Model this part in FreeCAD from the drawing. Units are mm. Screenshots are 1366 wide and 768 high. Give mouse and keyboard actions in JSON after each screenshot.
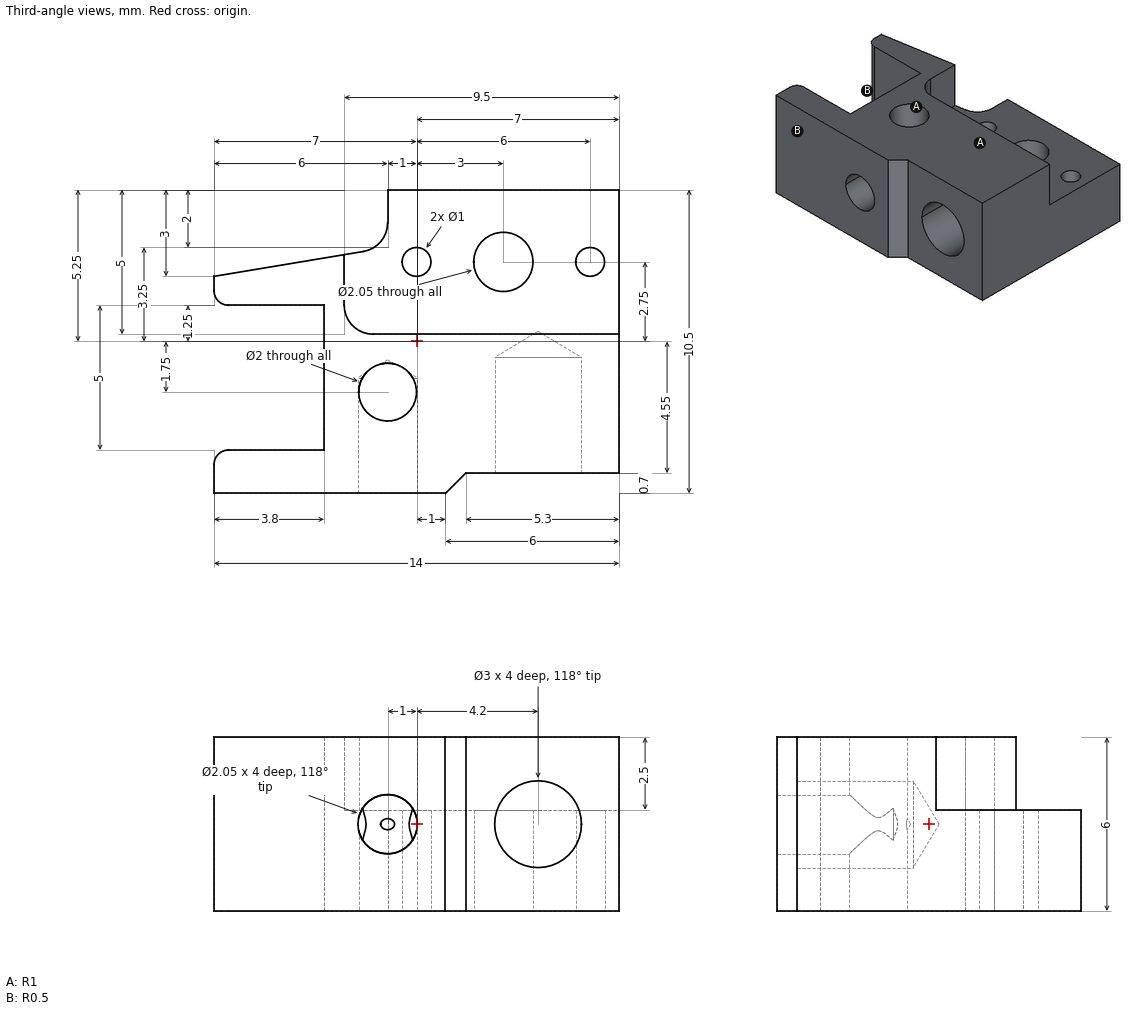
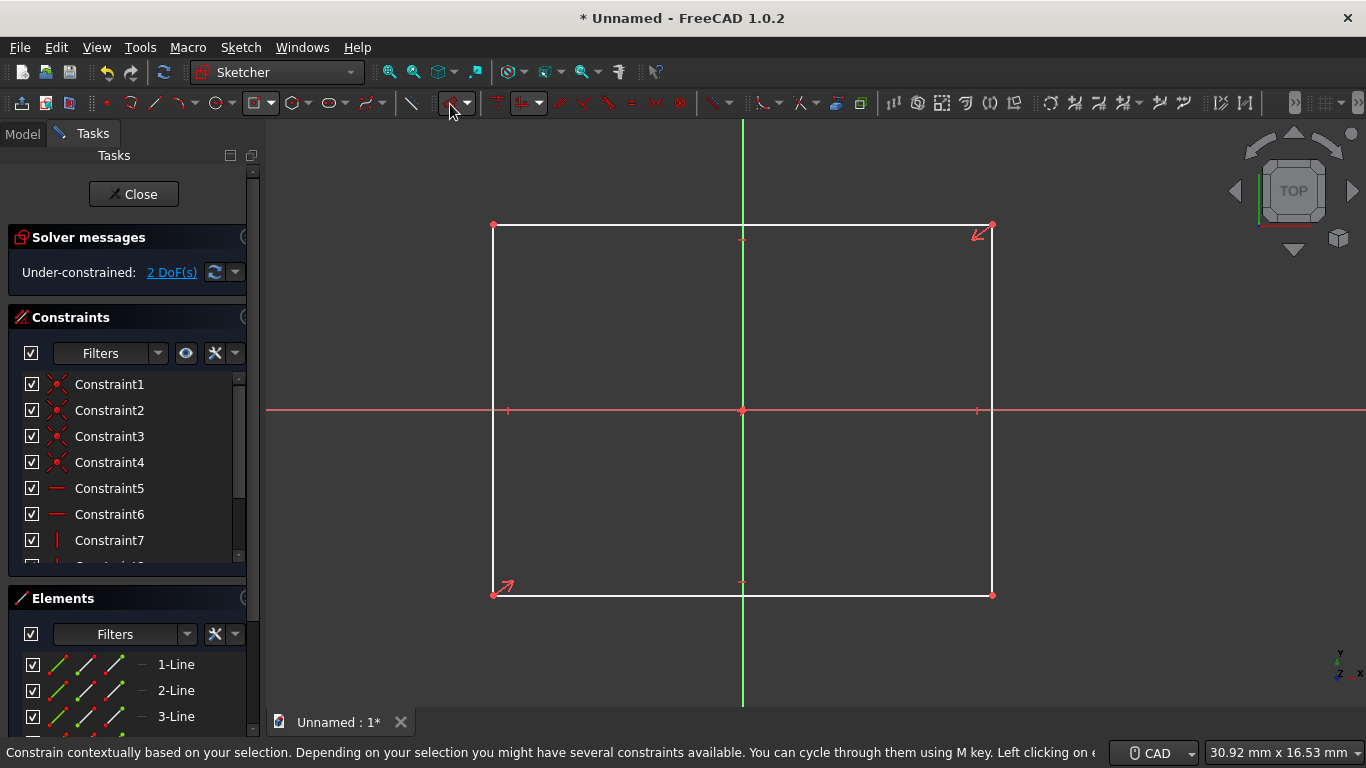
{"action": "left_click", "coordinate": [643, 596]}
{"action": "left_click", "coordinate": [628, 630]}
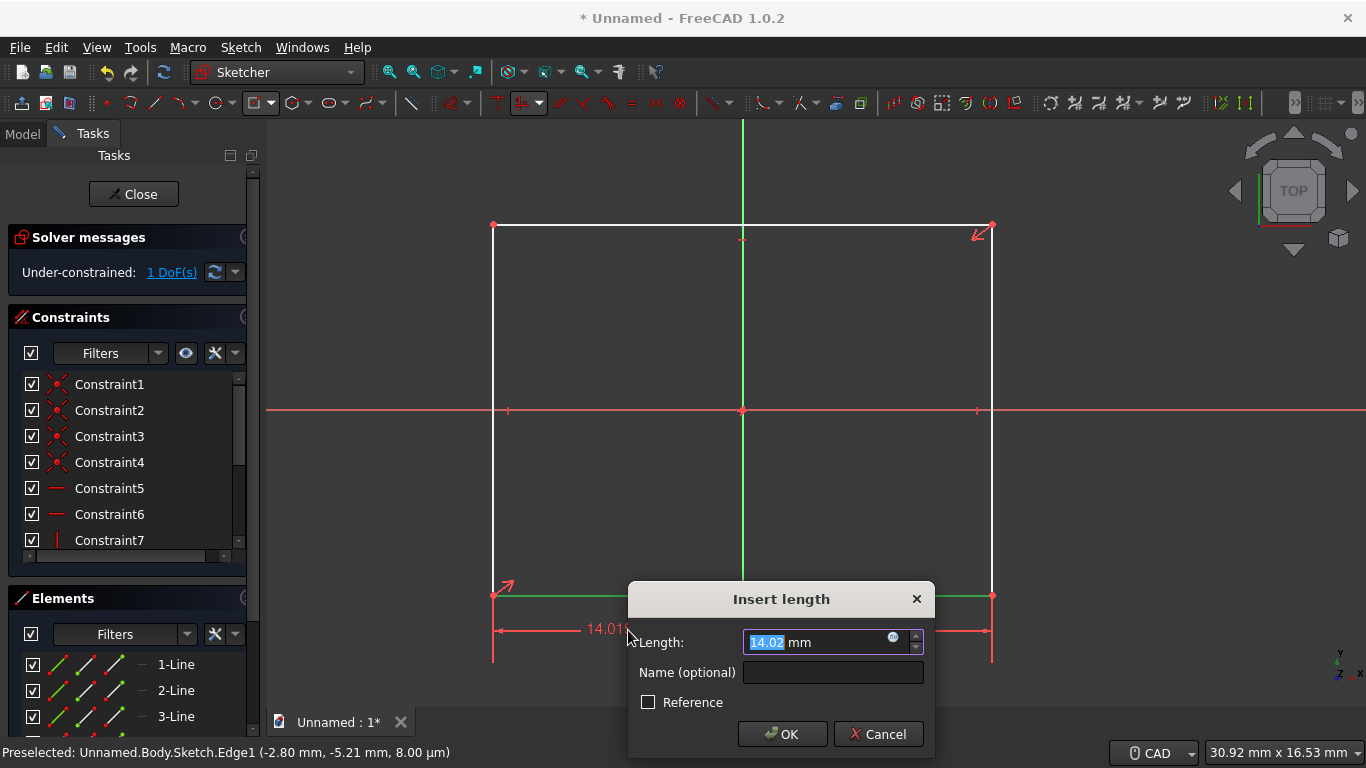
{"action": "type", "text": "14"}
{"action": "key", "text": "Return"}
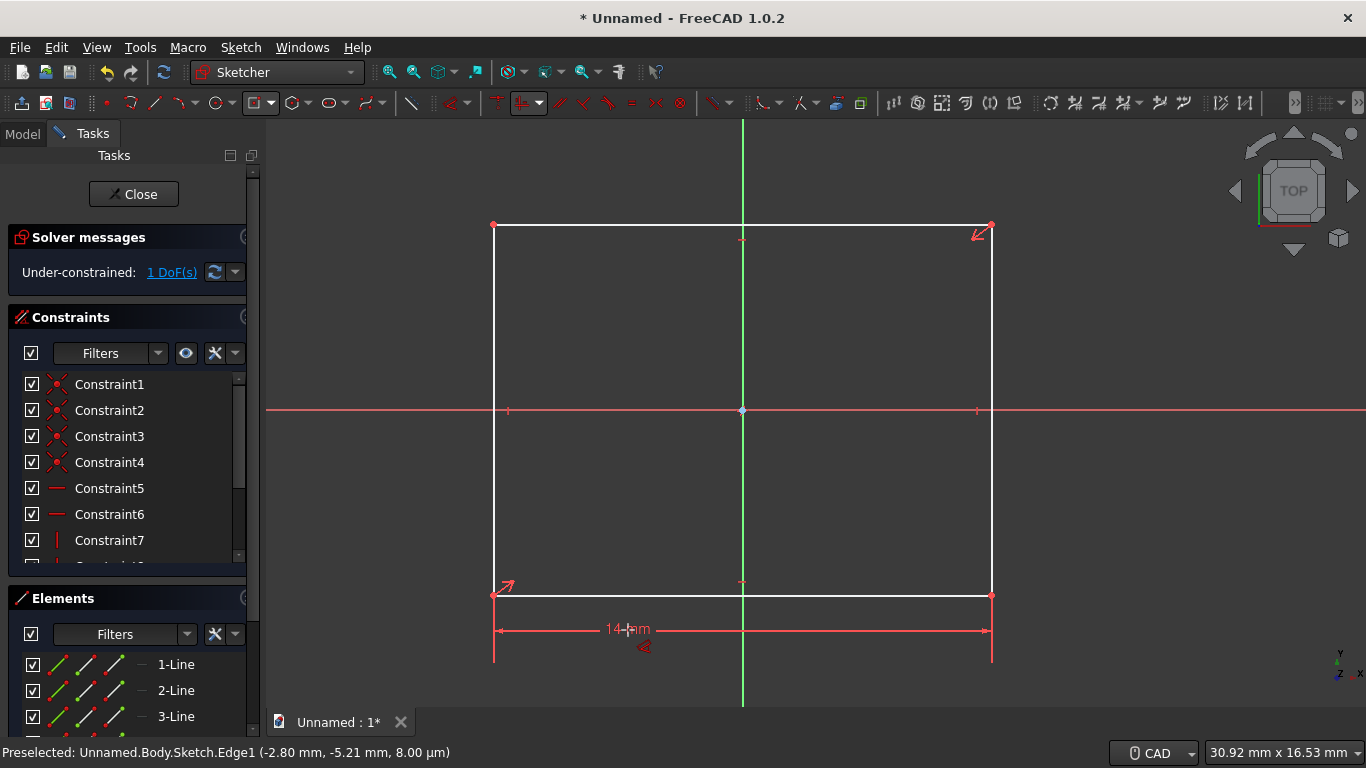
{"action": "left_click", "coordinate": [992, 485]}
{"action": "left_click", "coordinate": [1026, 325]}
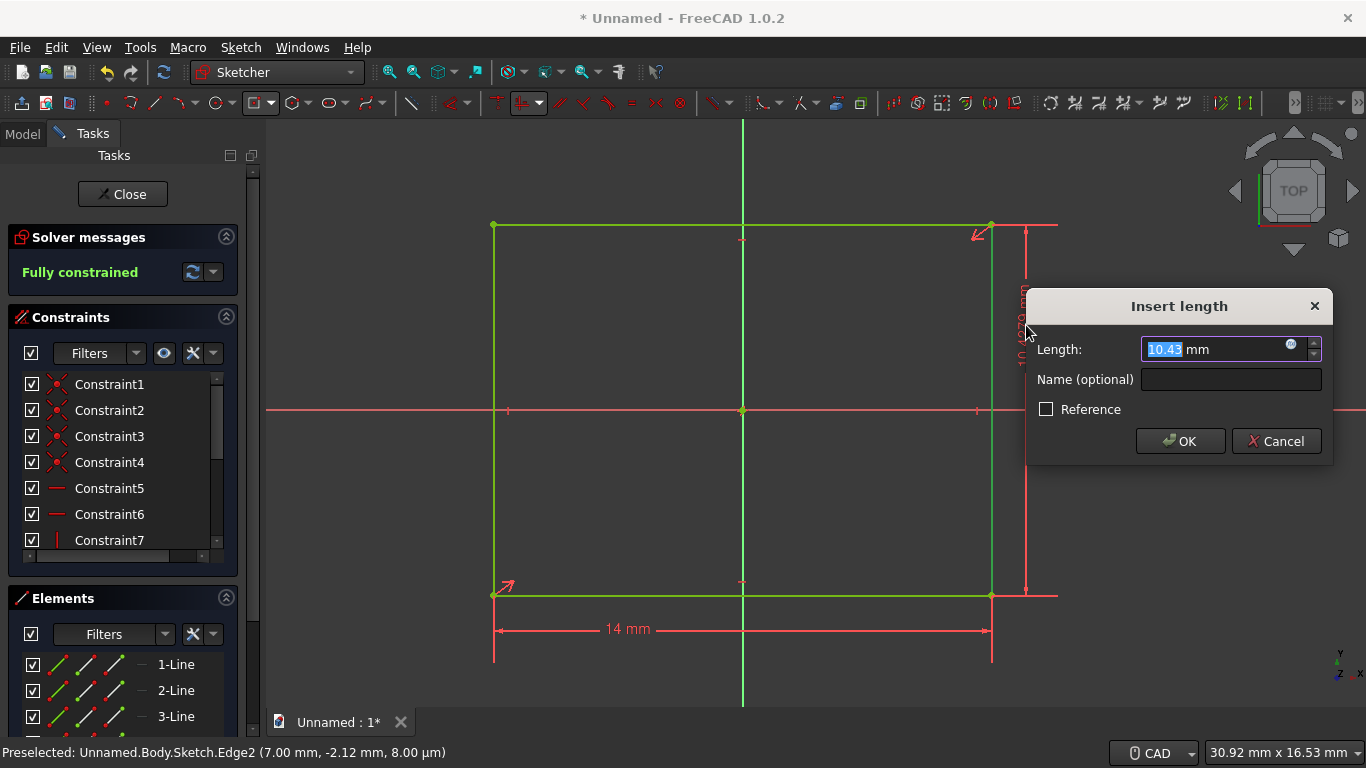
{"action": "type", "text": "10.5"}
{"action": "key", "text": "Return"}
{"action": "key", "text": "Escape"}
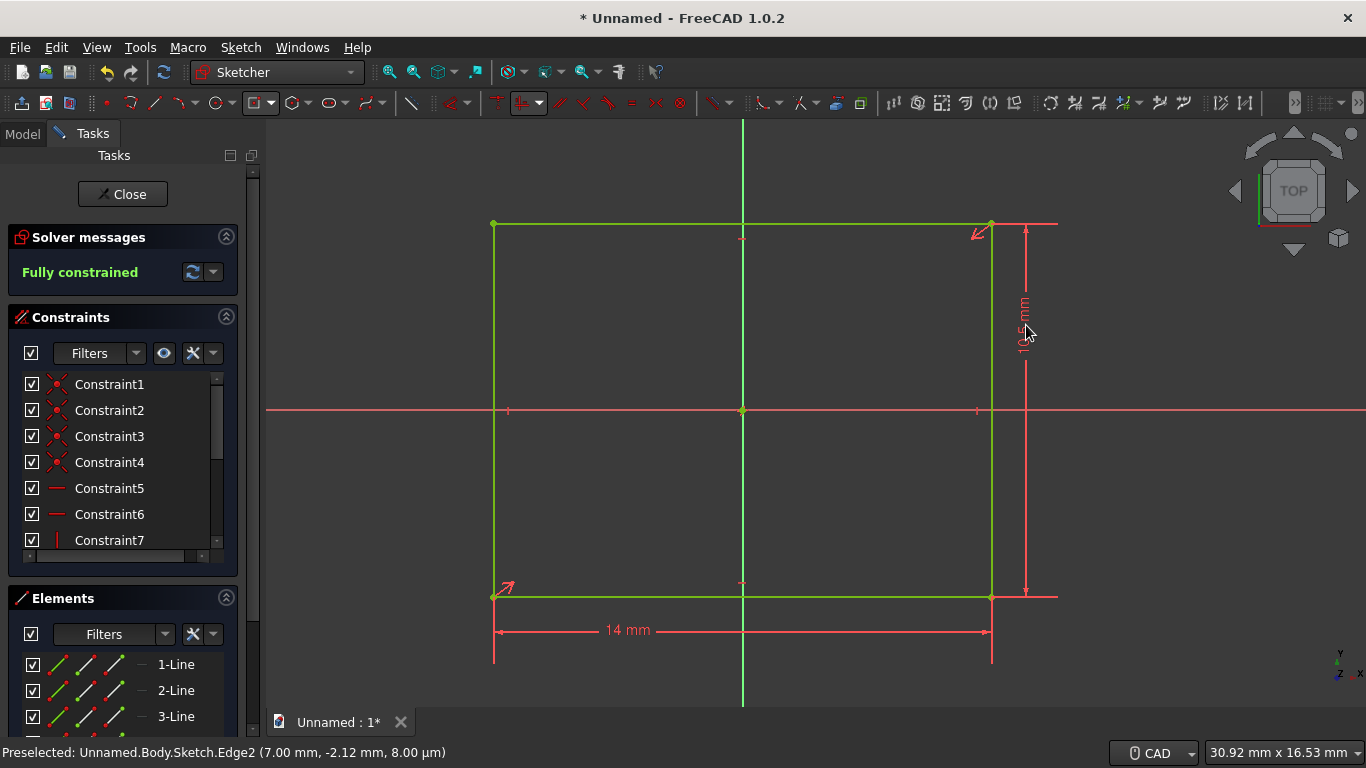
{"action": "left_click", "coordinate": [123, 194]}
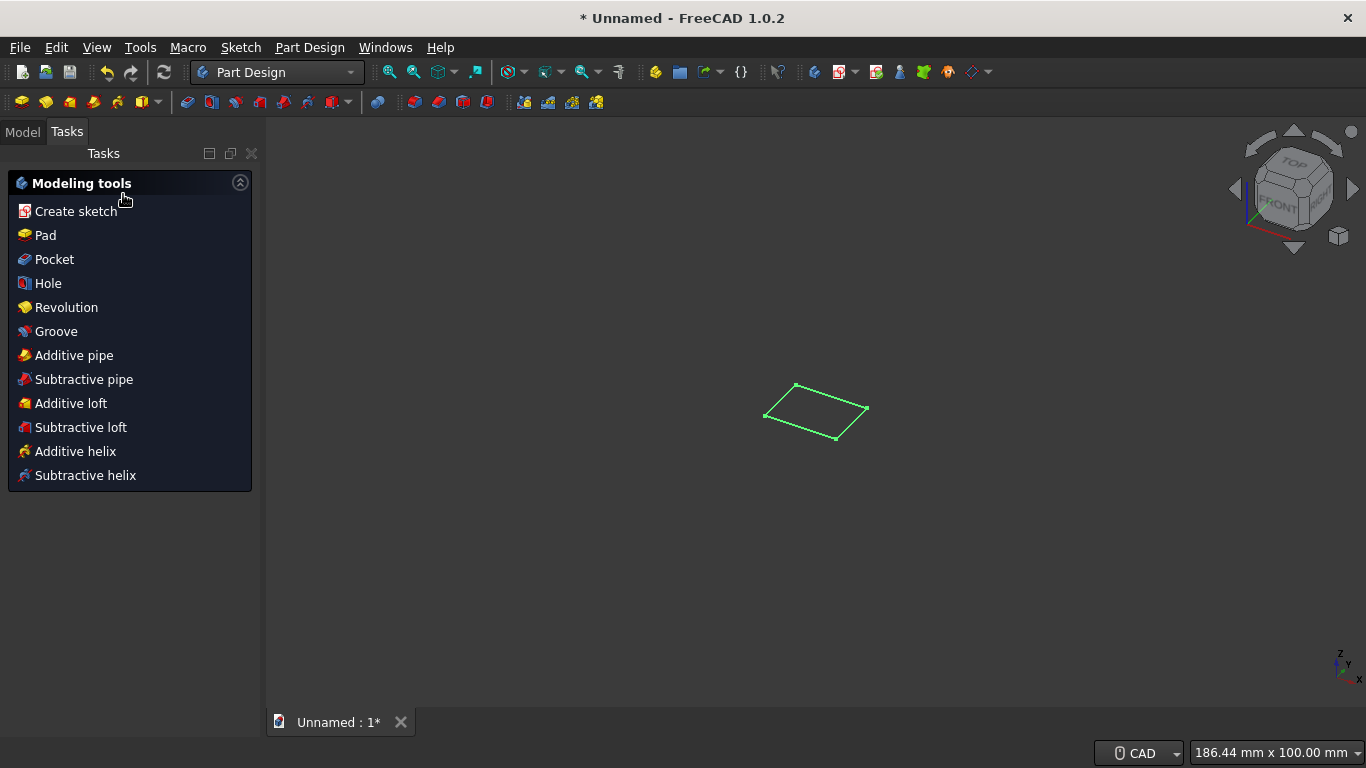
{"action": "left_click", "coordinate": [22, 102]}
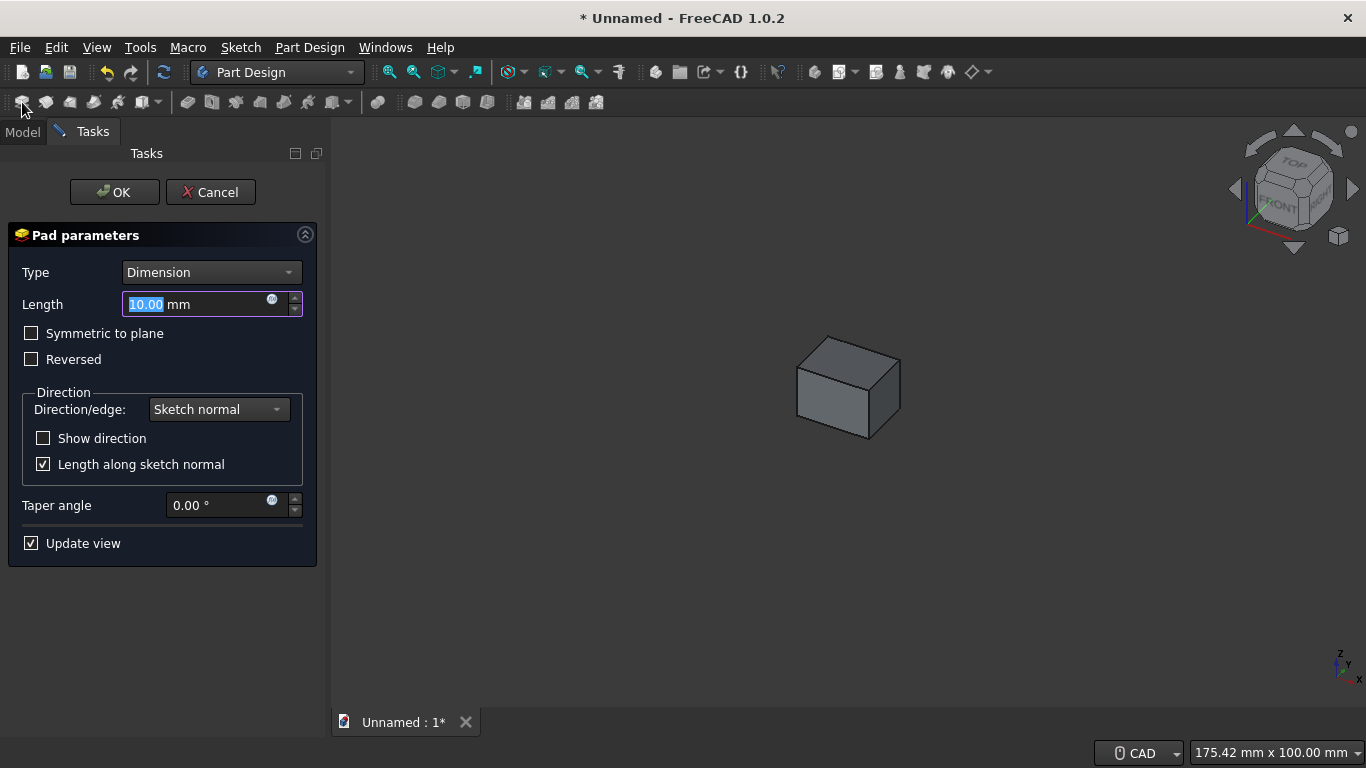
{"action": "type", "text": "6"}
{"action": "key", "text": "Tab"}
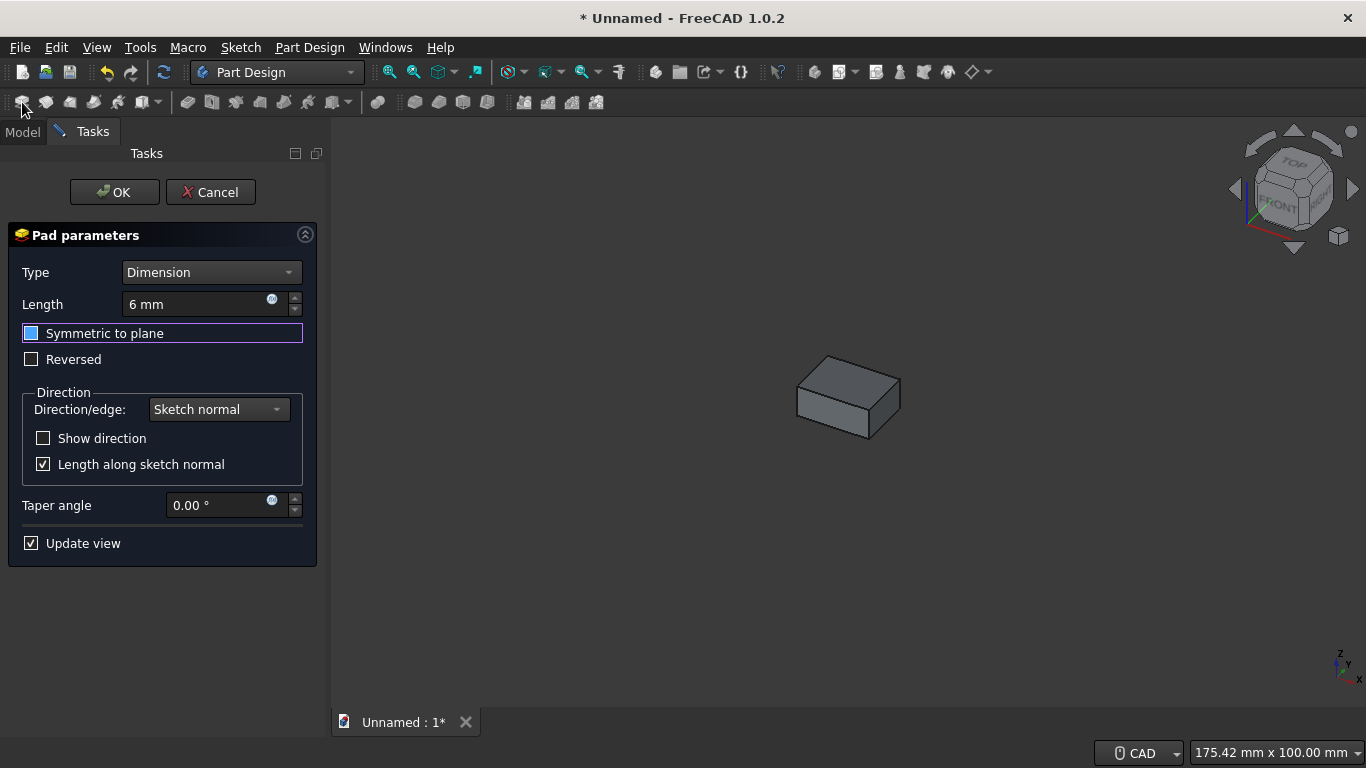
{"action": "left_click", "coordinate": [30, 333]}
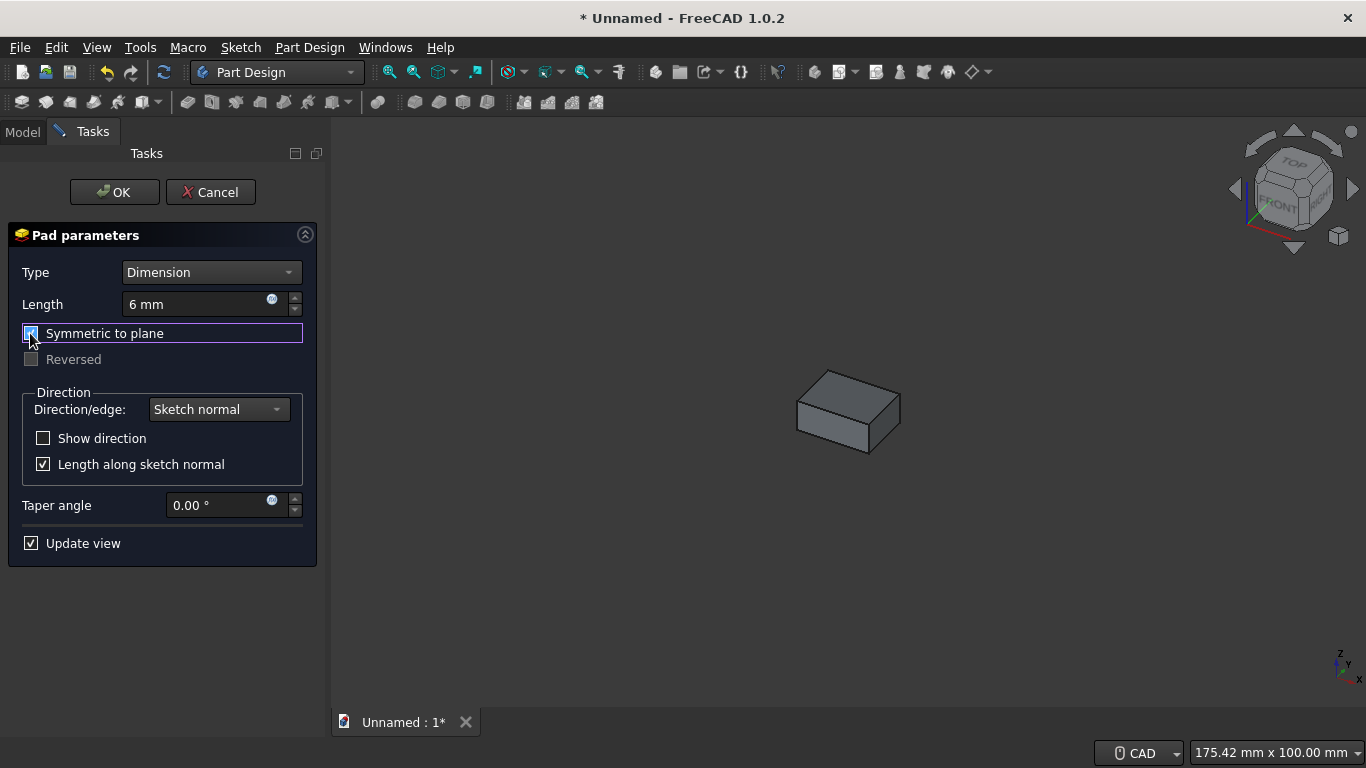
{"action": "left_click", "coordinate": [115, 192]}